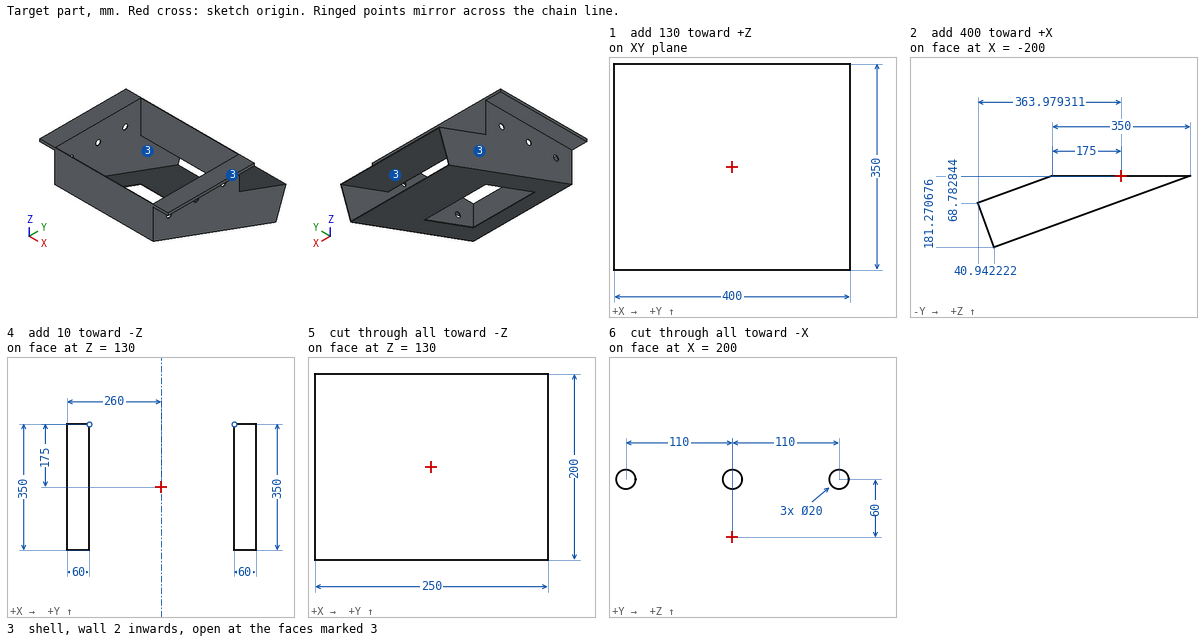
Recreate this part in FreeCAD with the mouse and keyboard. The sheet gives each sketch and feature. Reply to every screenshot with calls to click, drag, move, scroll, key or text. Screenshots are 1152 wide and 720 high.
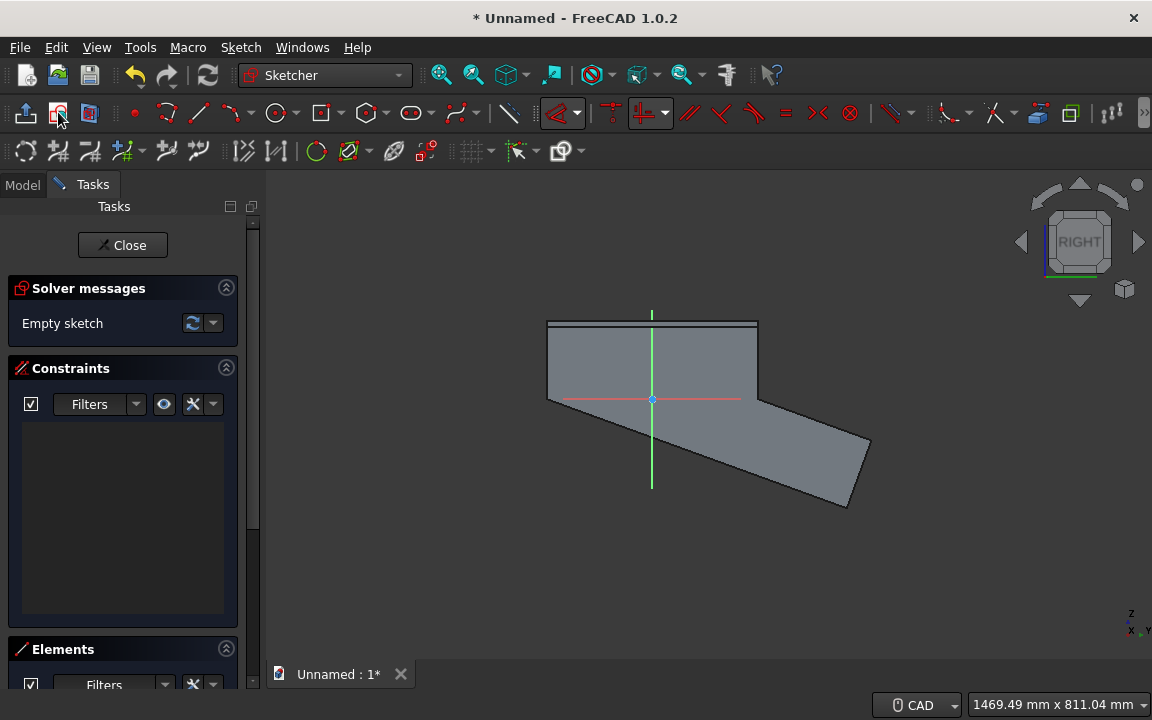
click(90, 114)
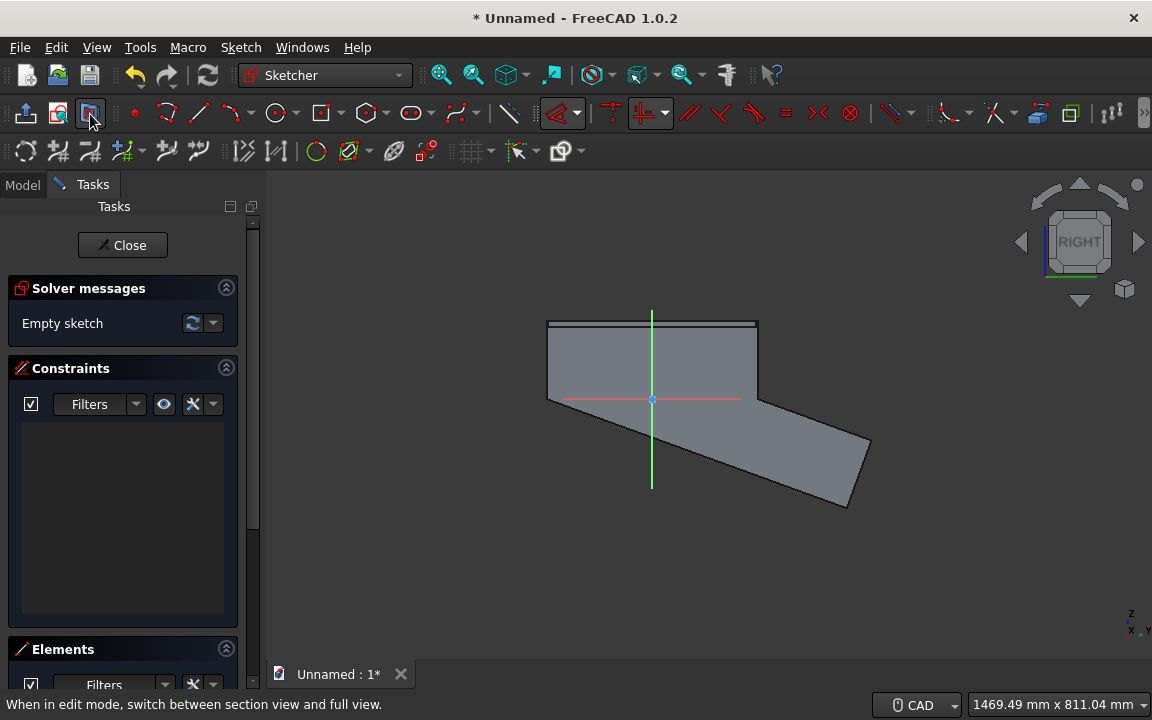
scroll(657, 362, up, 6)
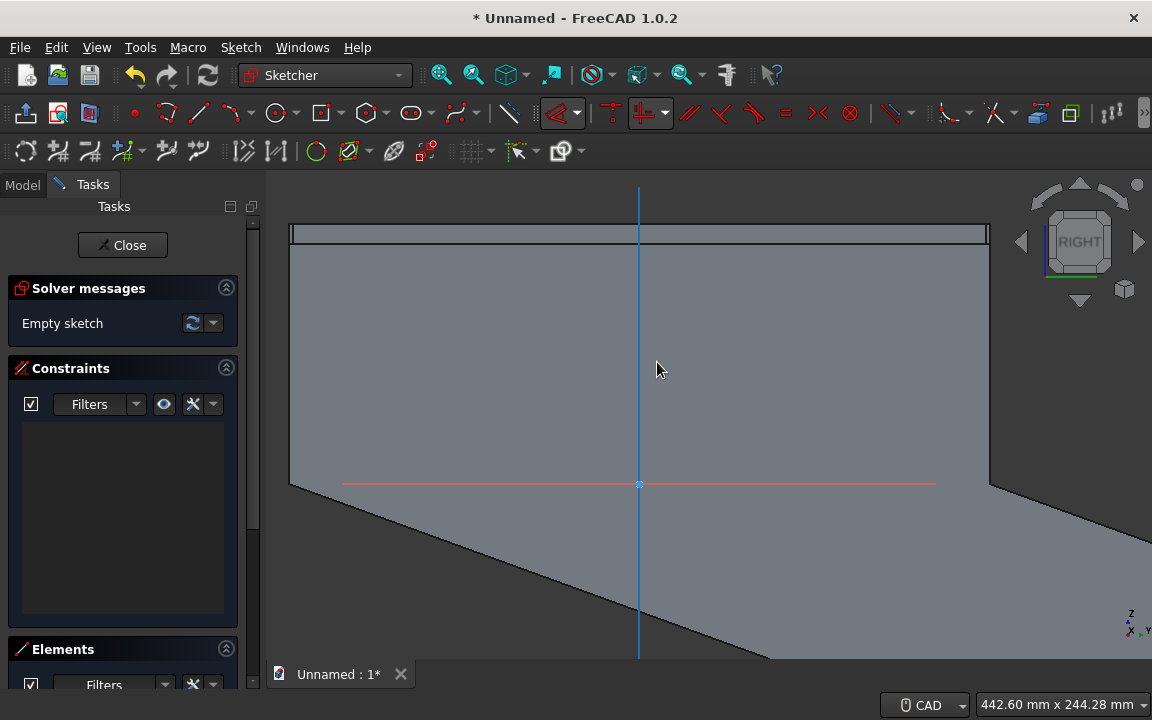
click(276, 114)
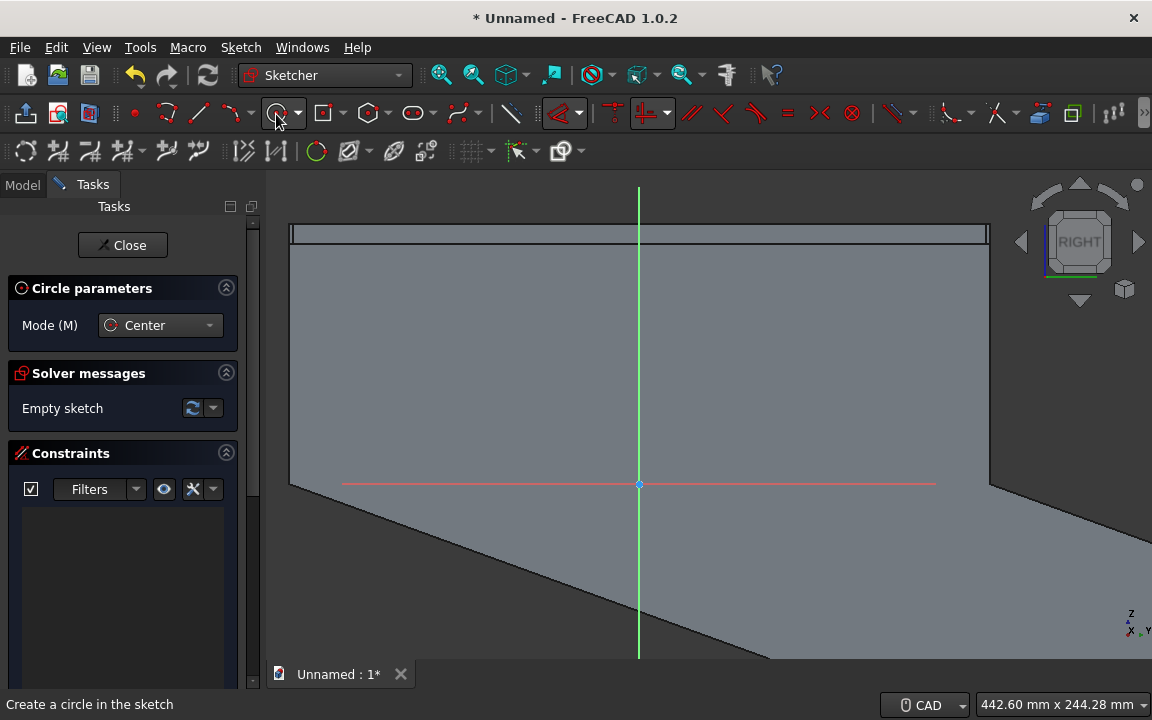
click(860, 364)
move(874, 350)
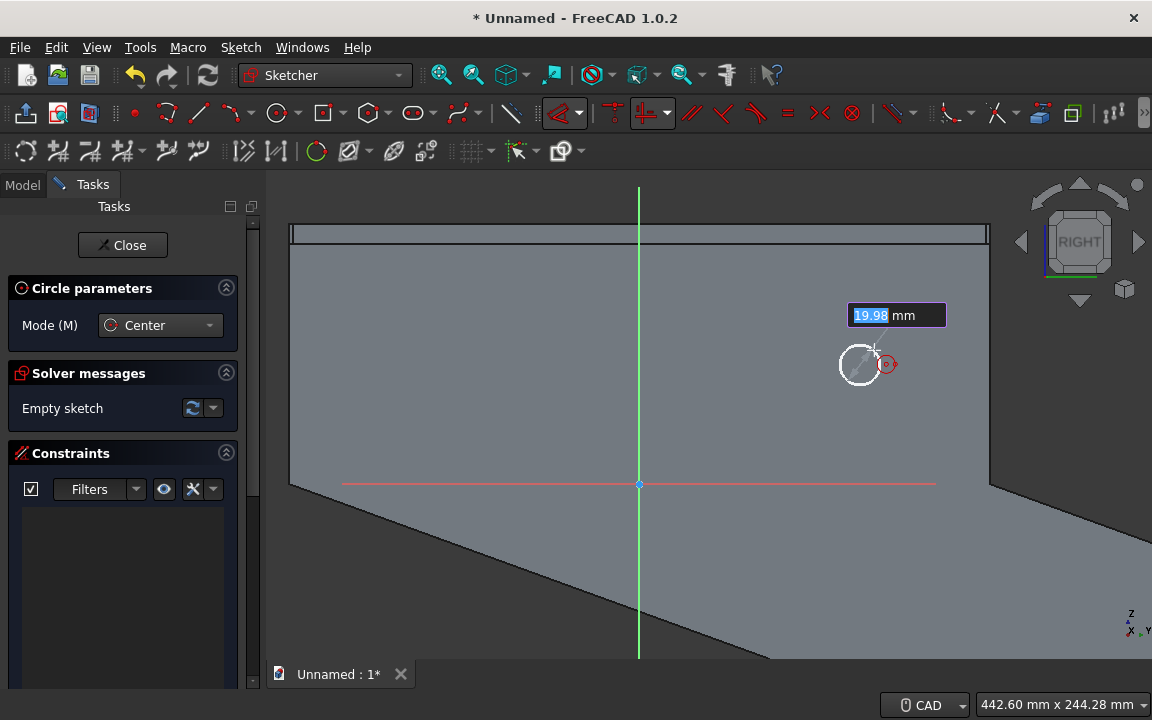
text(20)
key(Return)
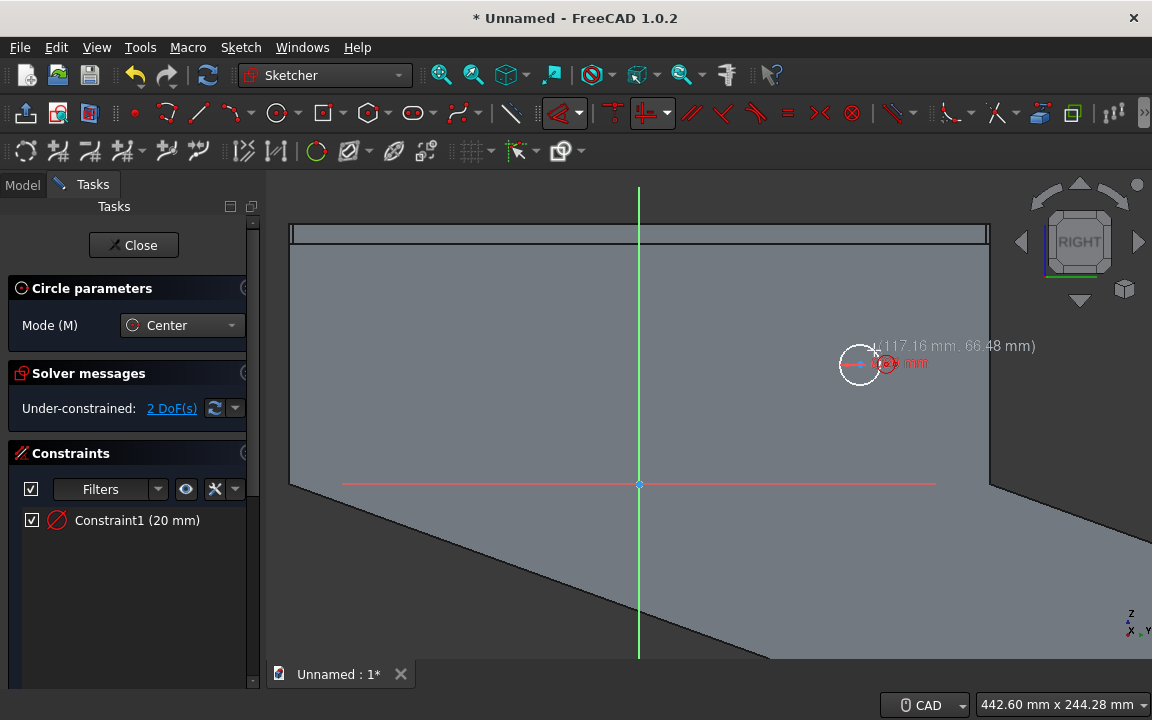
click(419, 364)
move(433, 350)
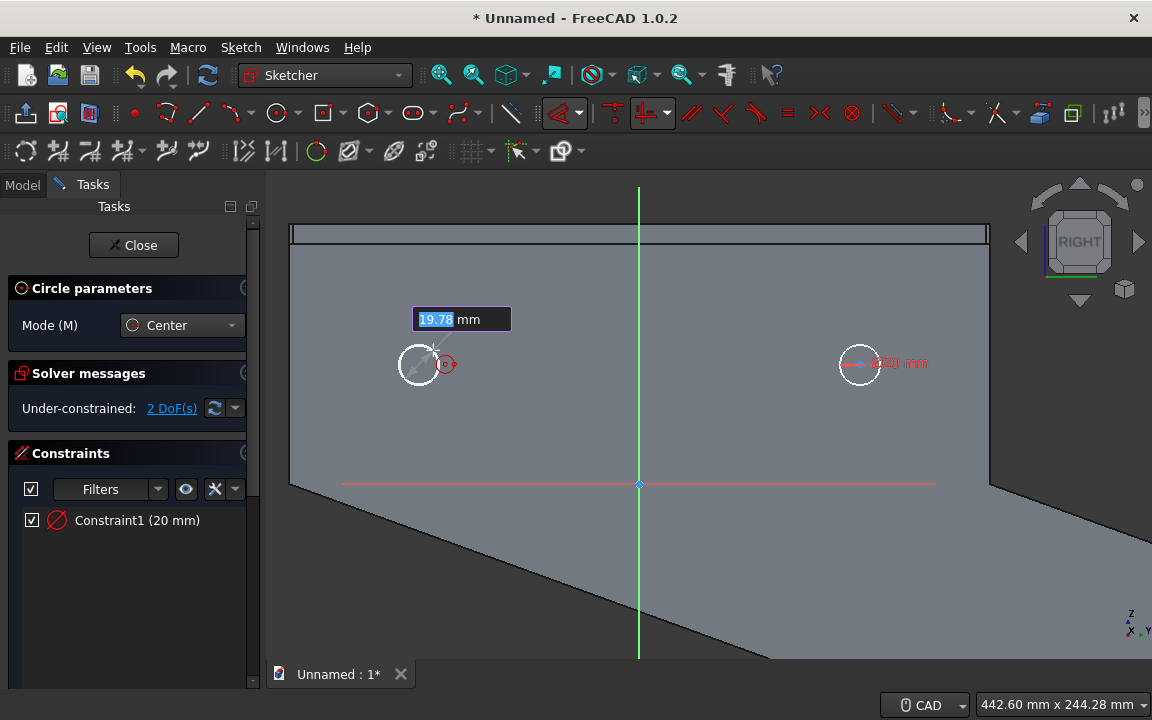
text(20)
key(Return)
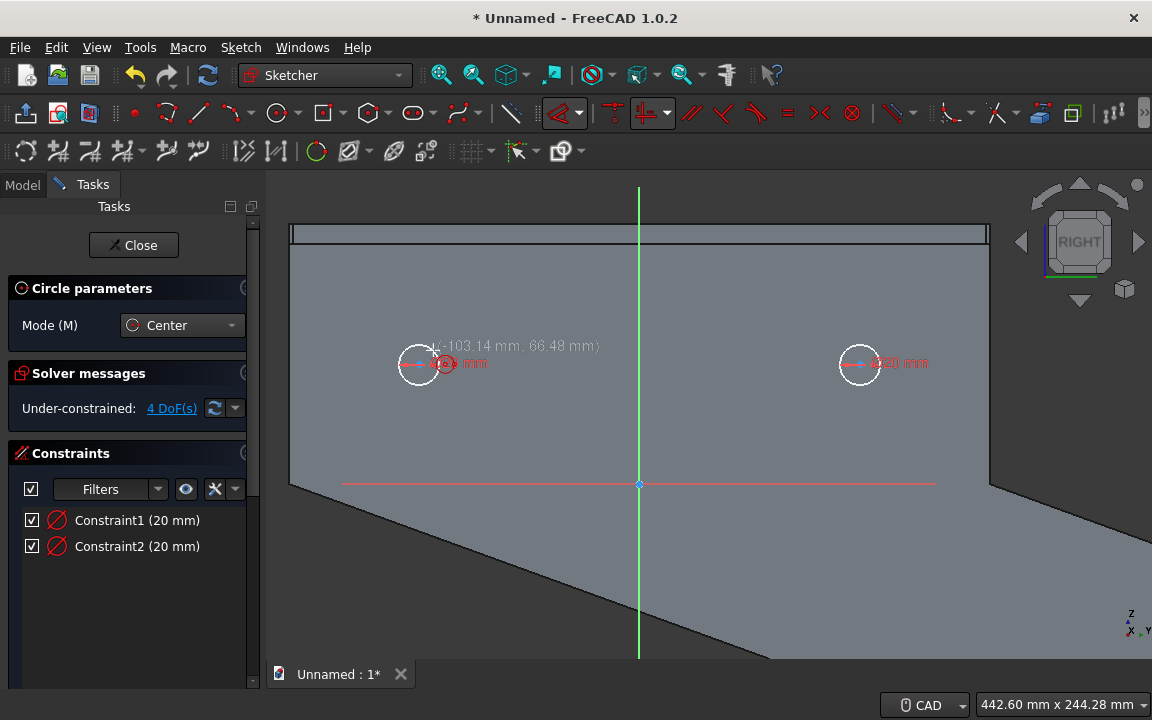
click(639, 364)
move(654, 350)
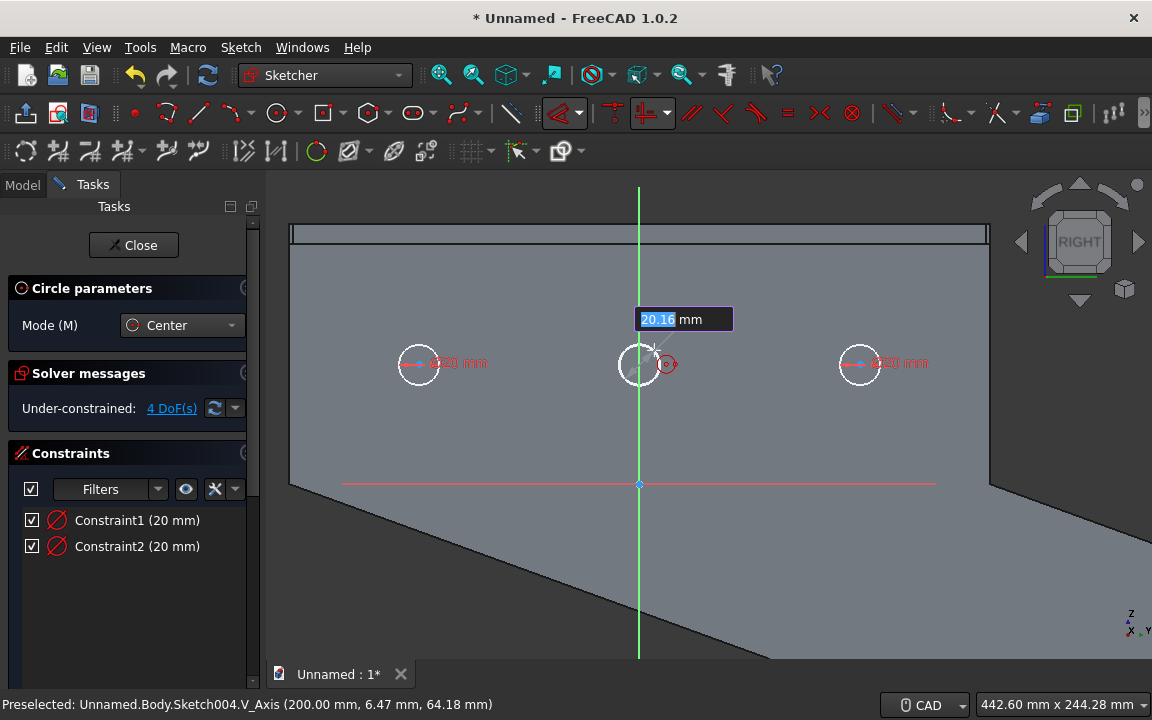
text(20)
key(Return)
key(Escape)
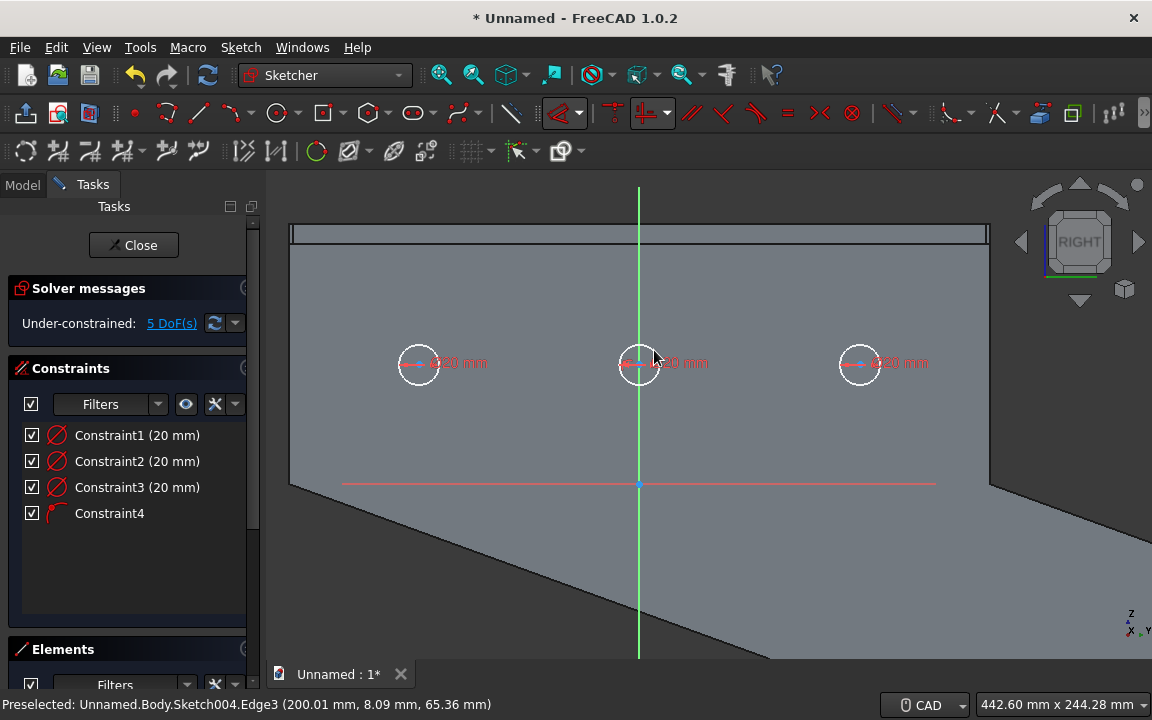
click(860, 365)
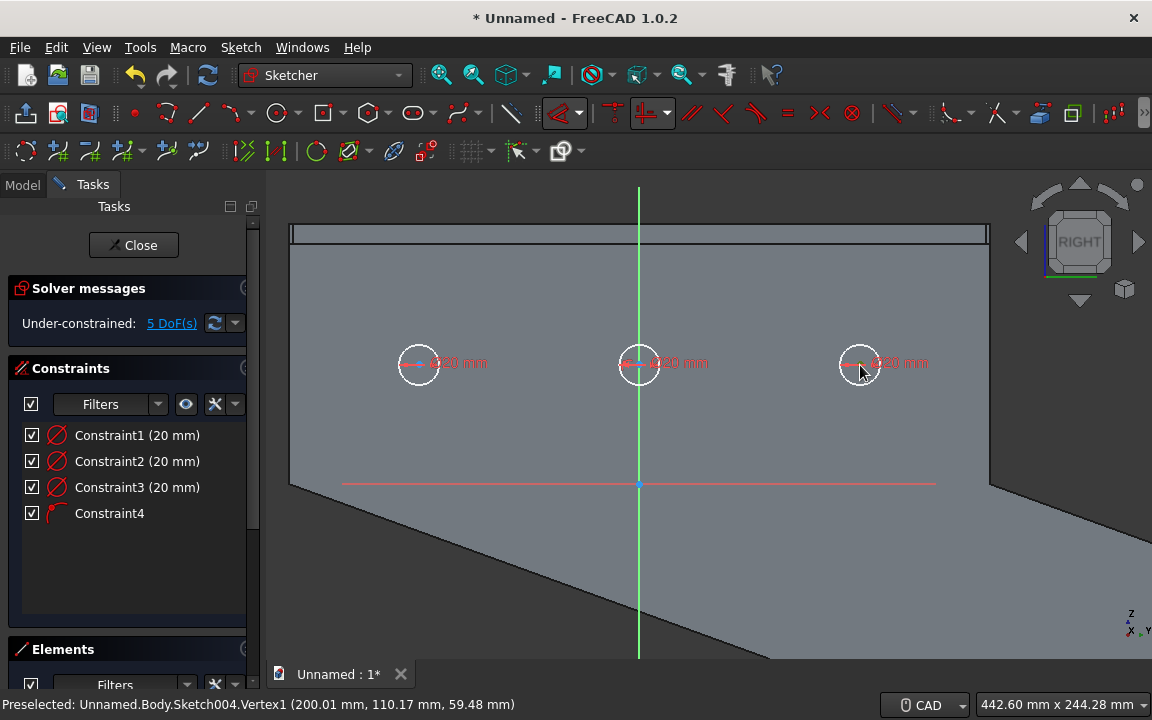
click(419, 365)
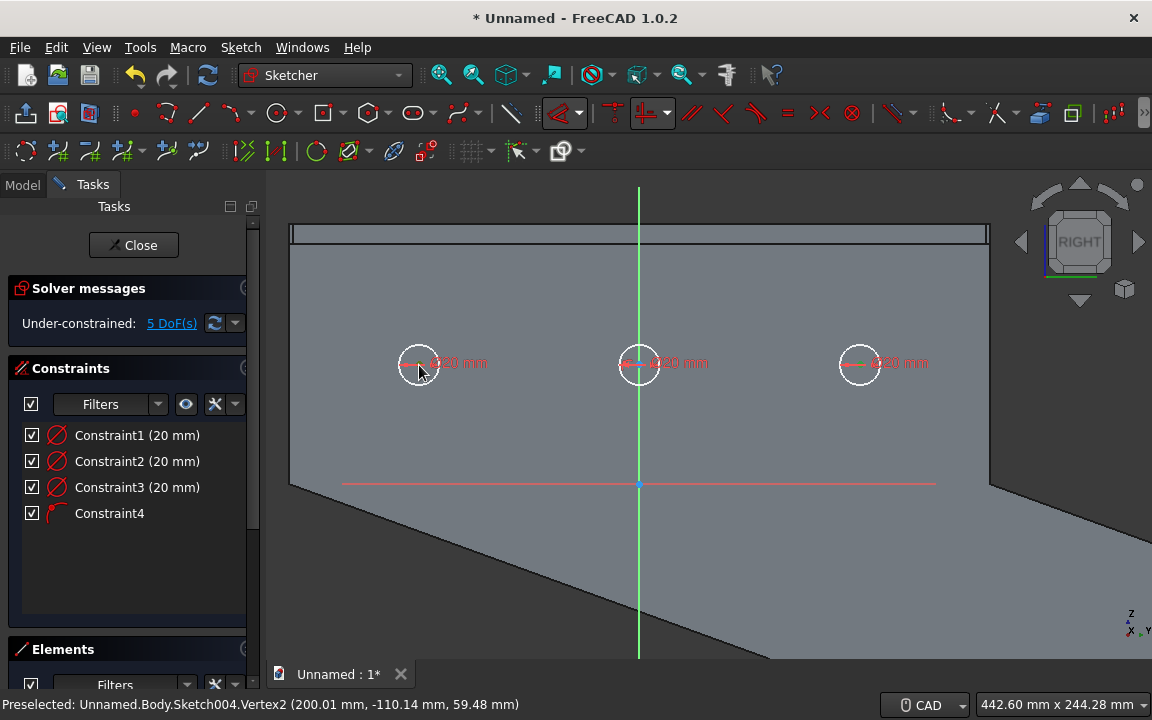
key(h)